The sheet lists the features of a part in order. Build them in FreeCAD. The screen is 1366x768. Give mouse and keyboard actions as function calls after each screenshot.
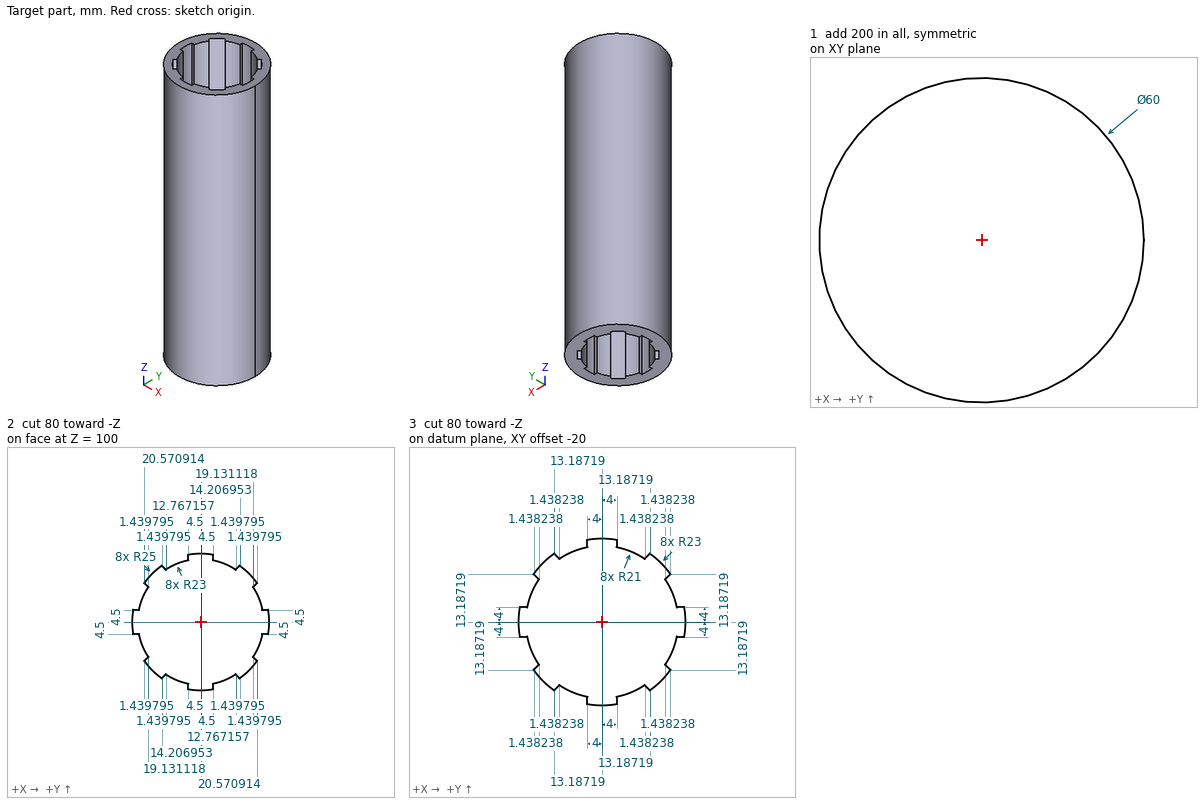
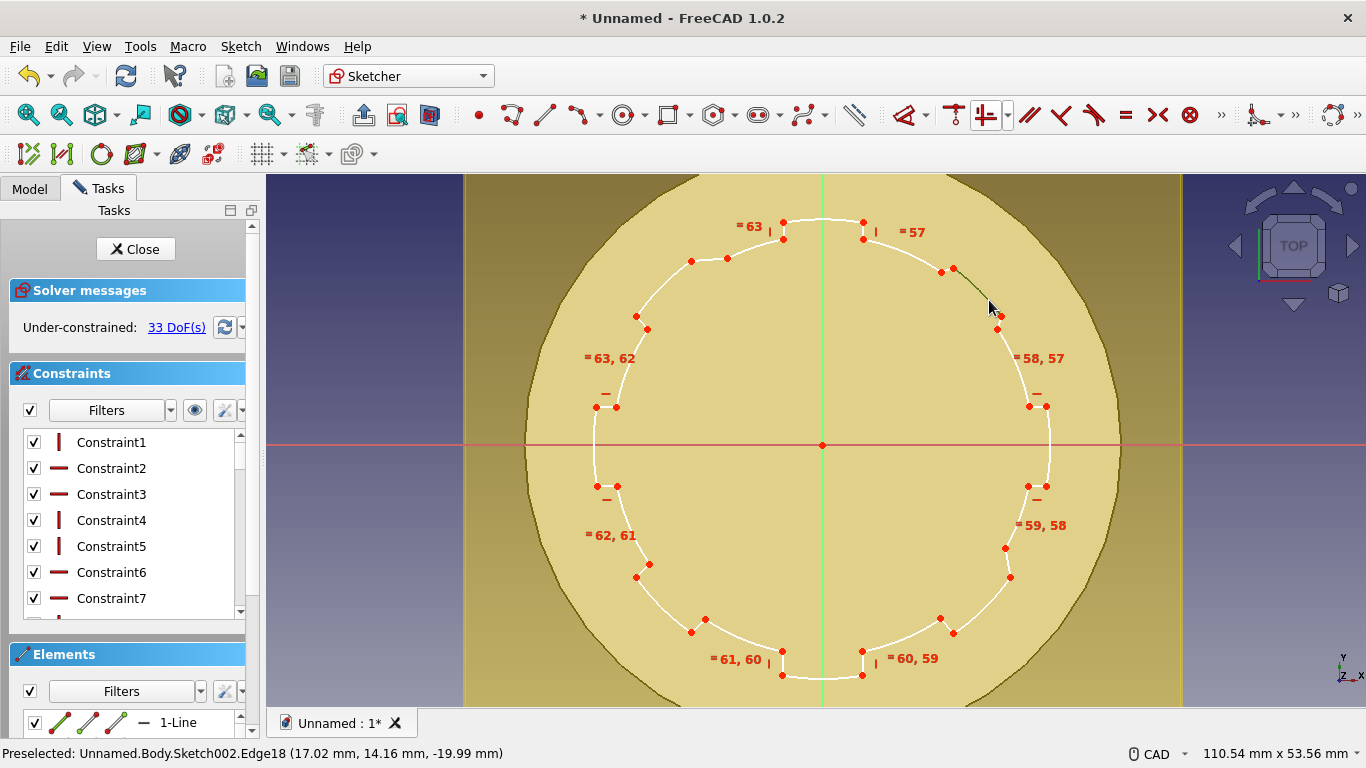
click(1050, 463)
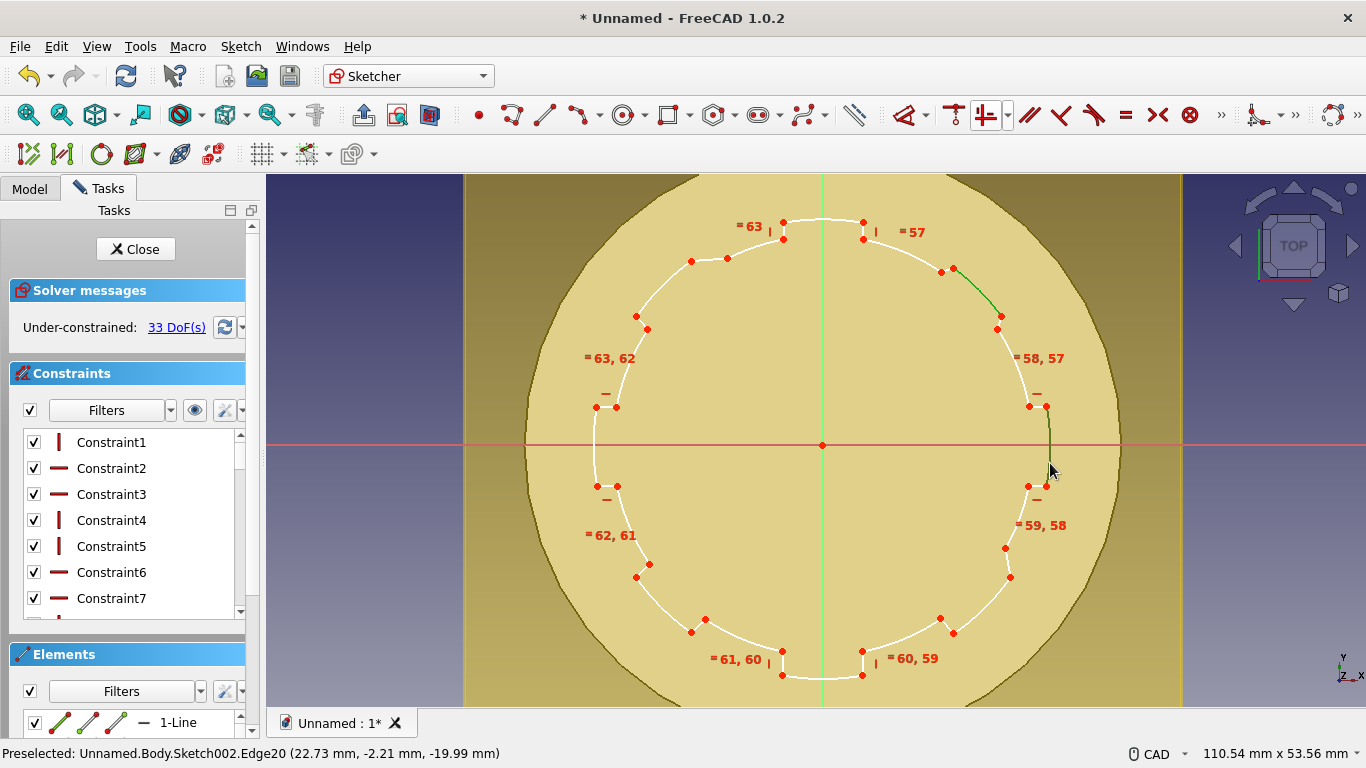
click(973, 619)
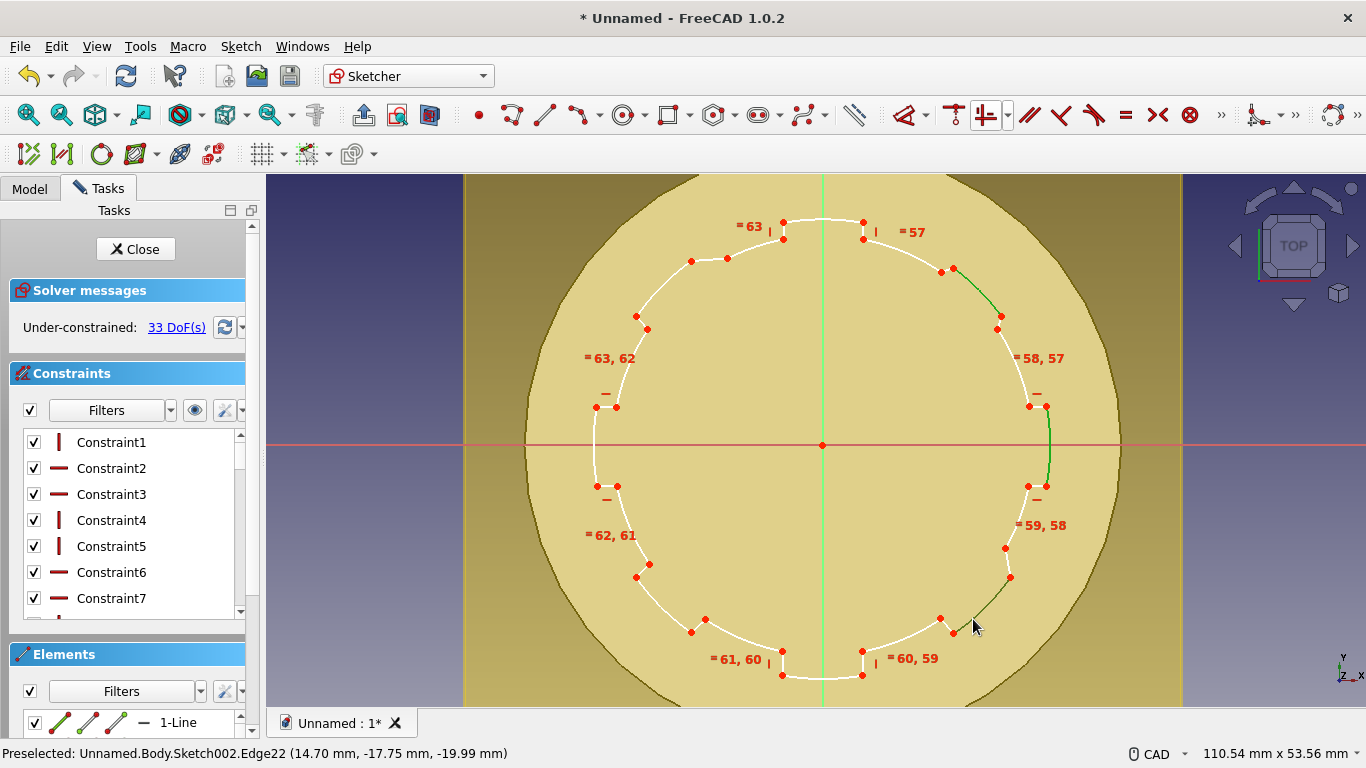
click(807, 678)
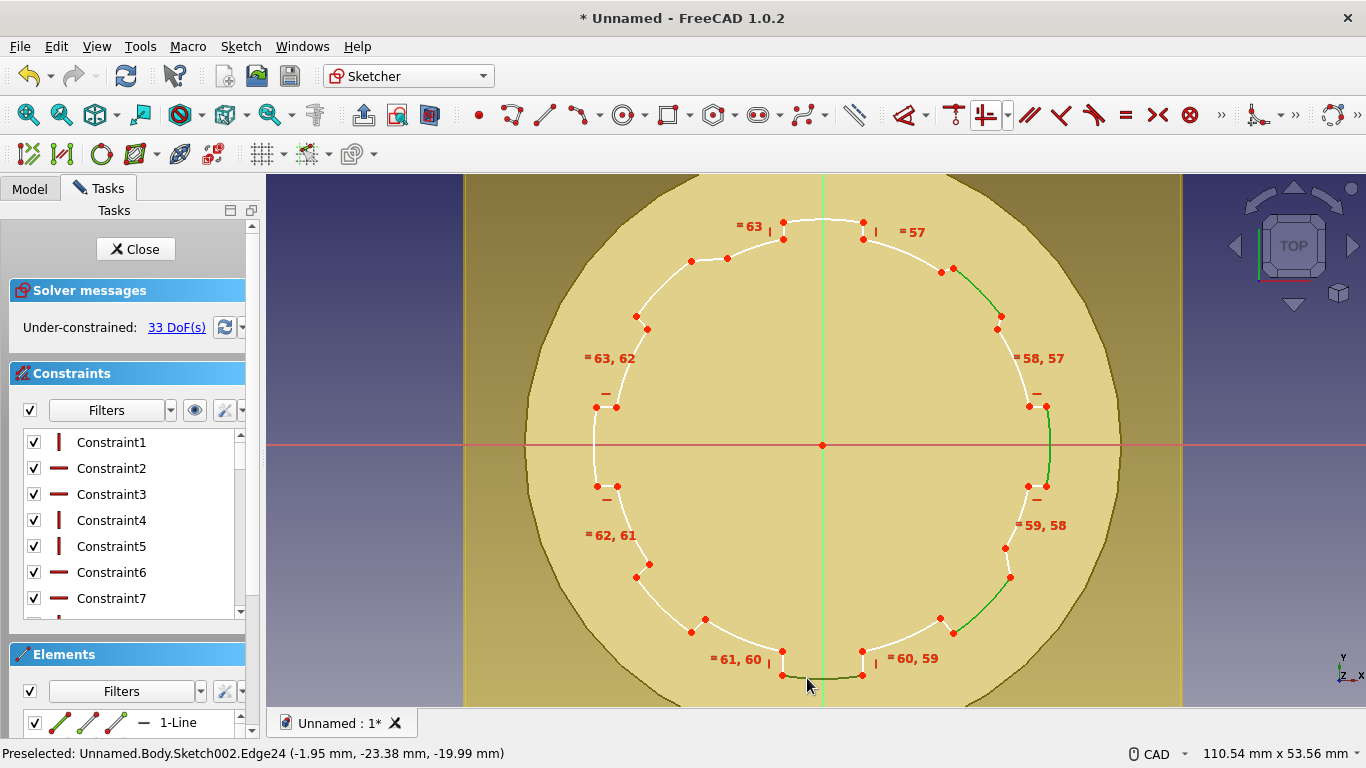
click(651, 596)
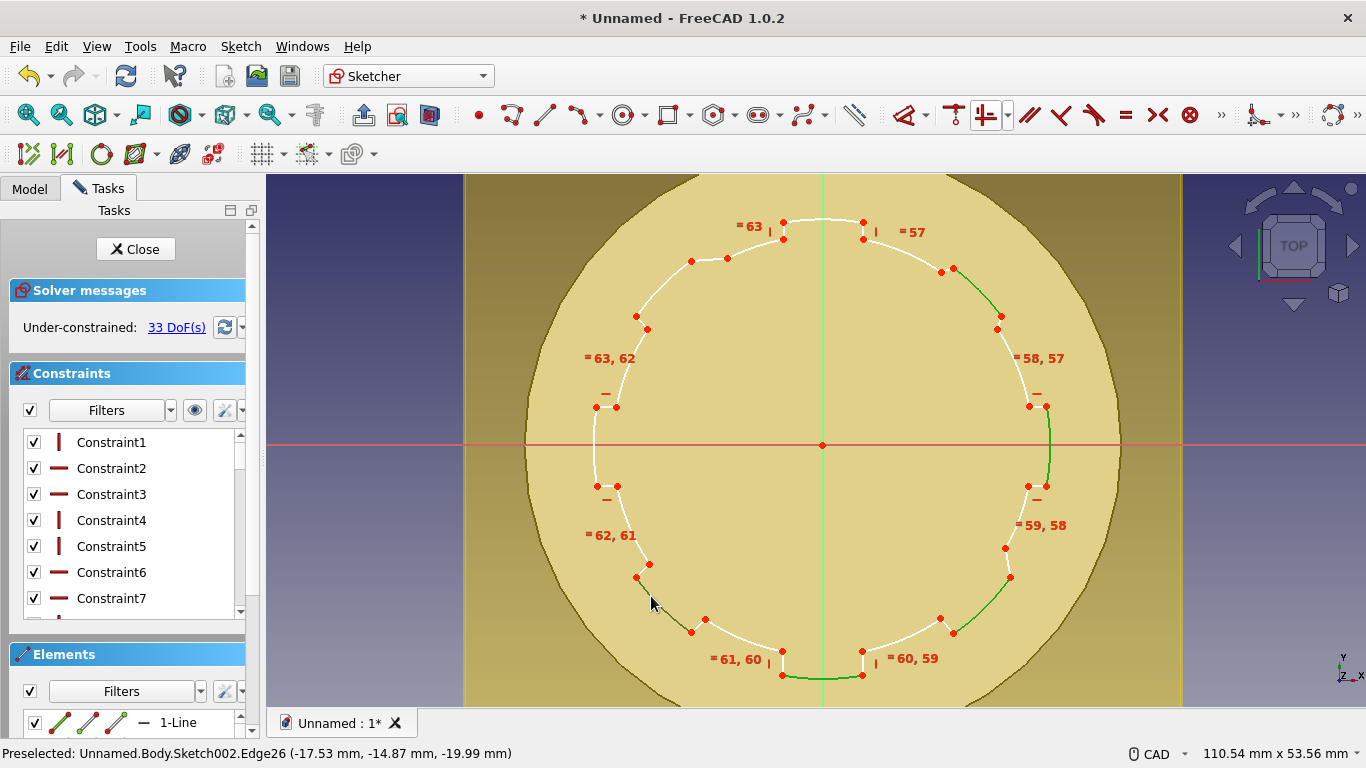
click(594, 431)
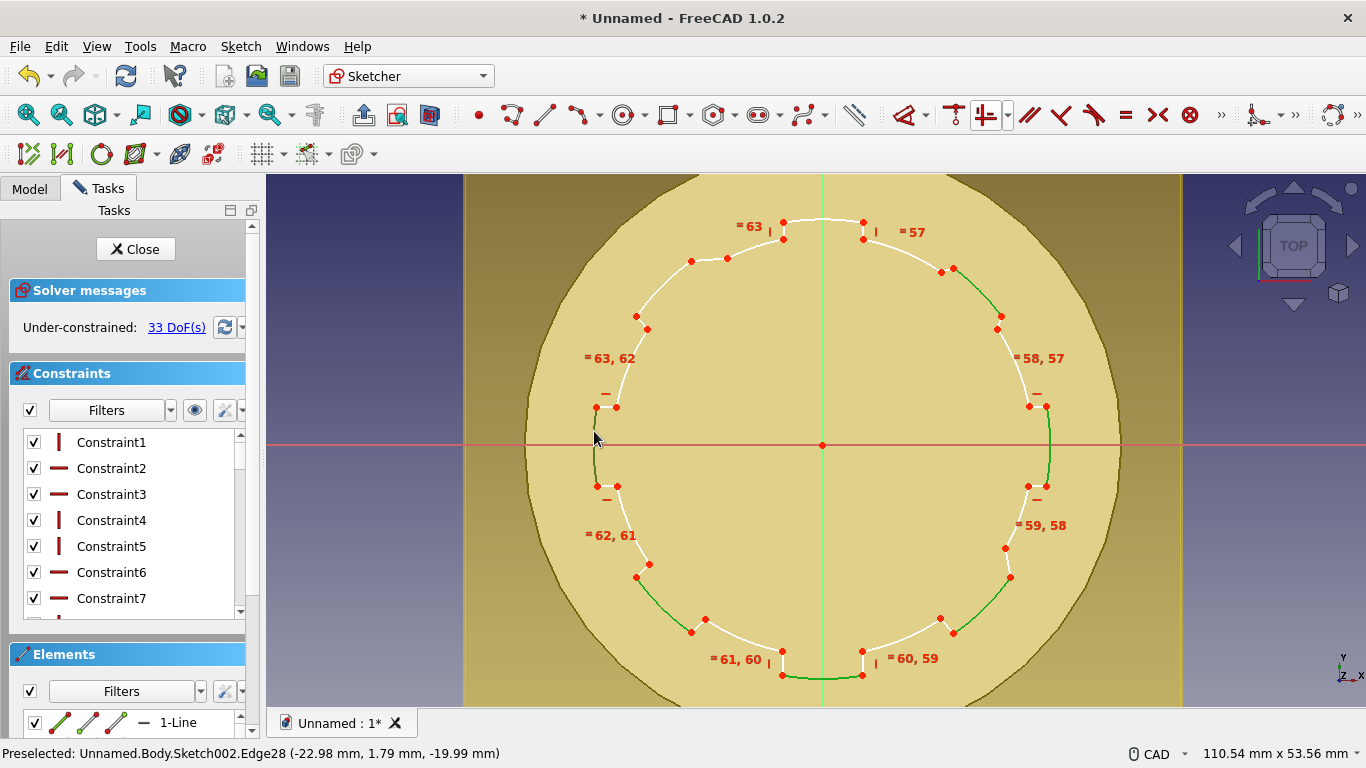
click(673, 276)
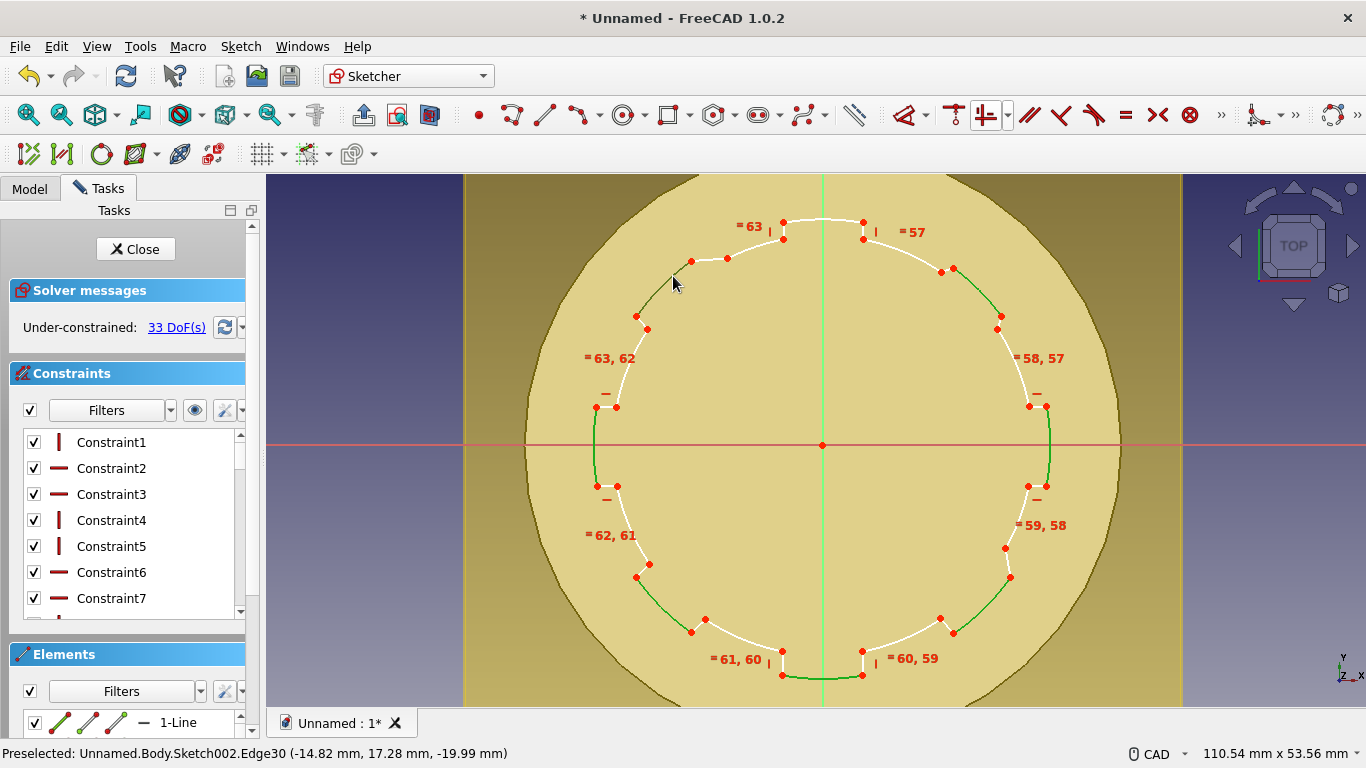
click(839, 220)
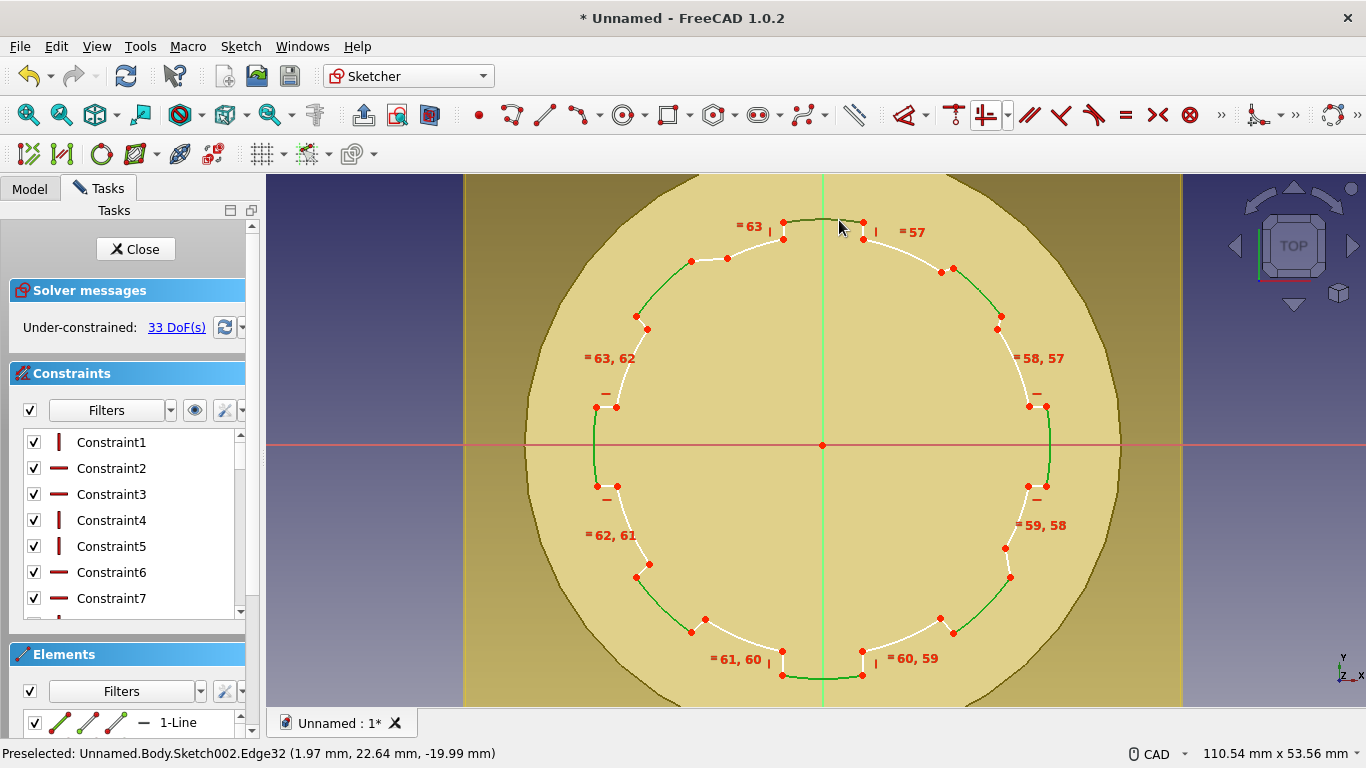
click(1126, 116)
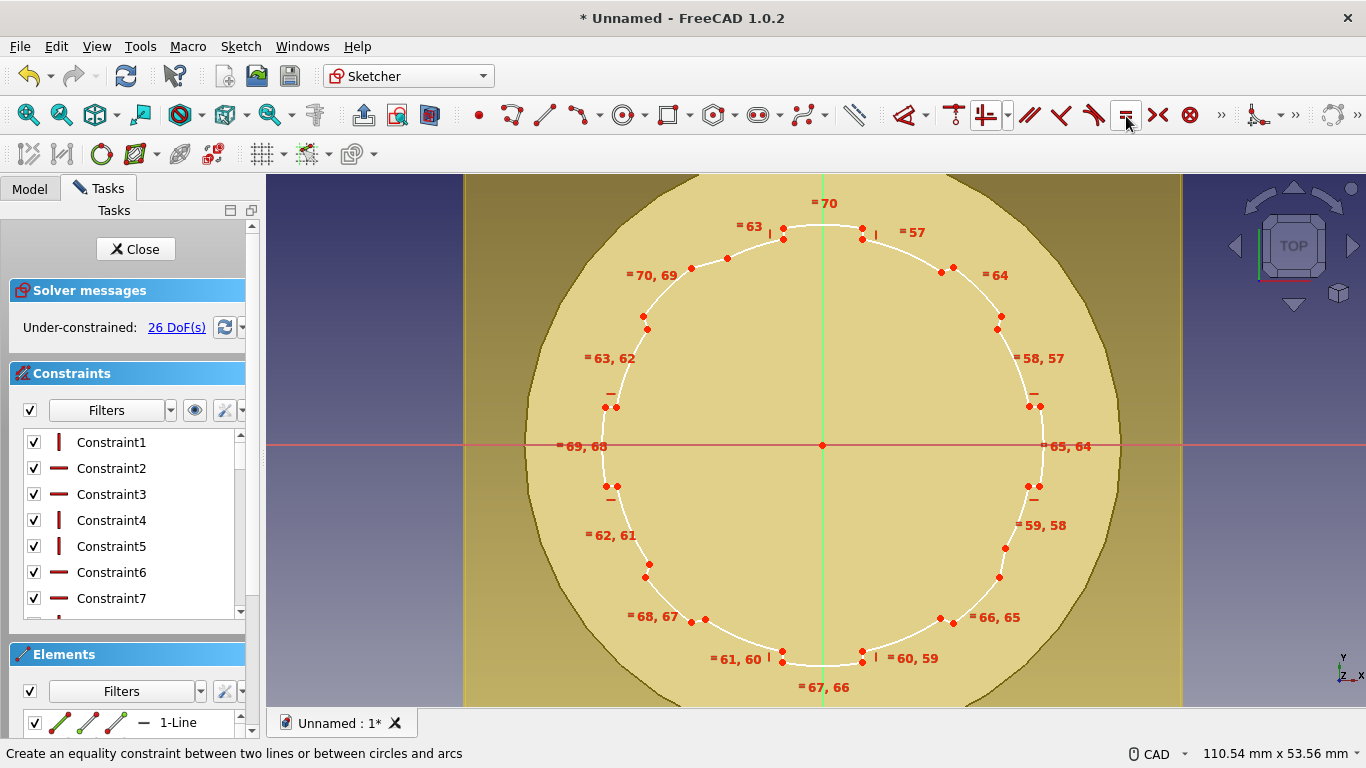
click(904, 116)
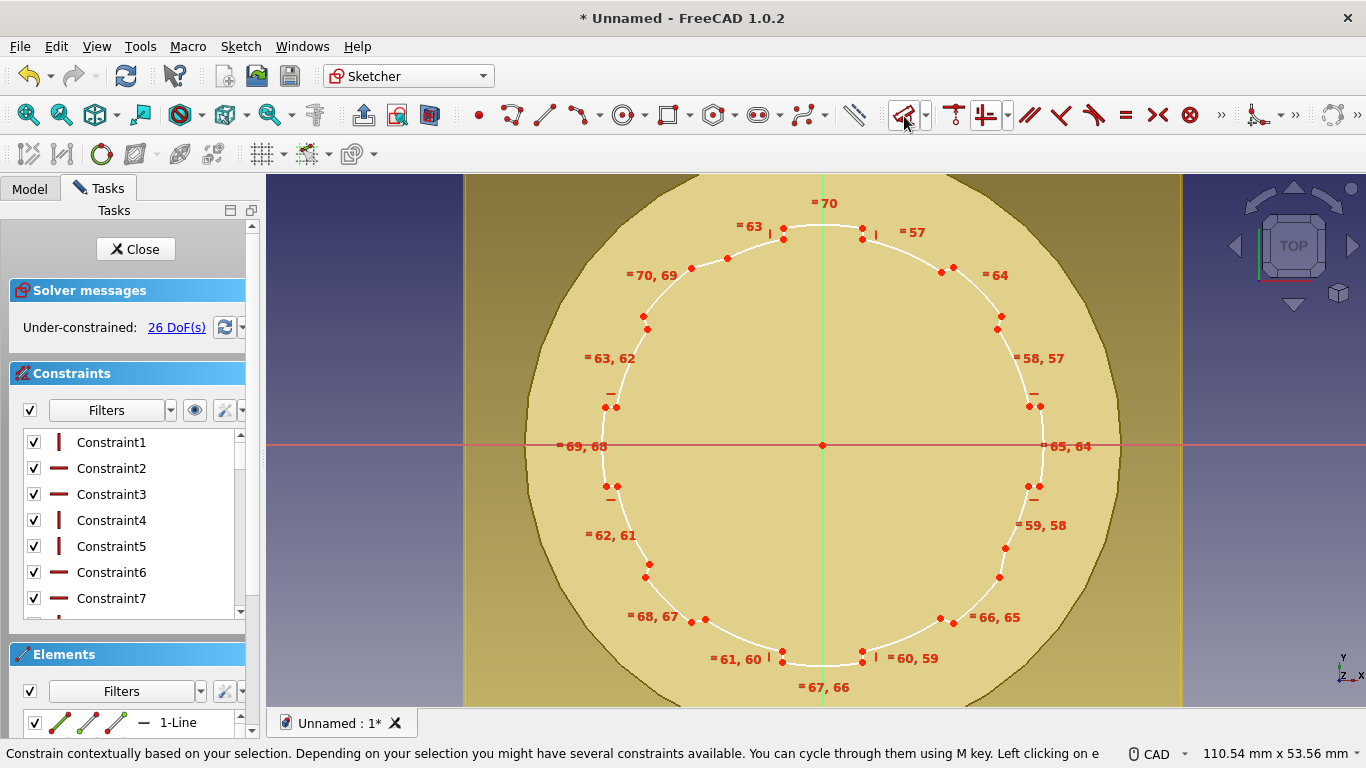
click(919, 259)
click(934, 231)